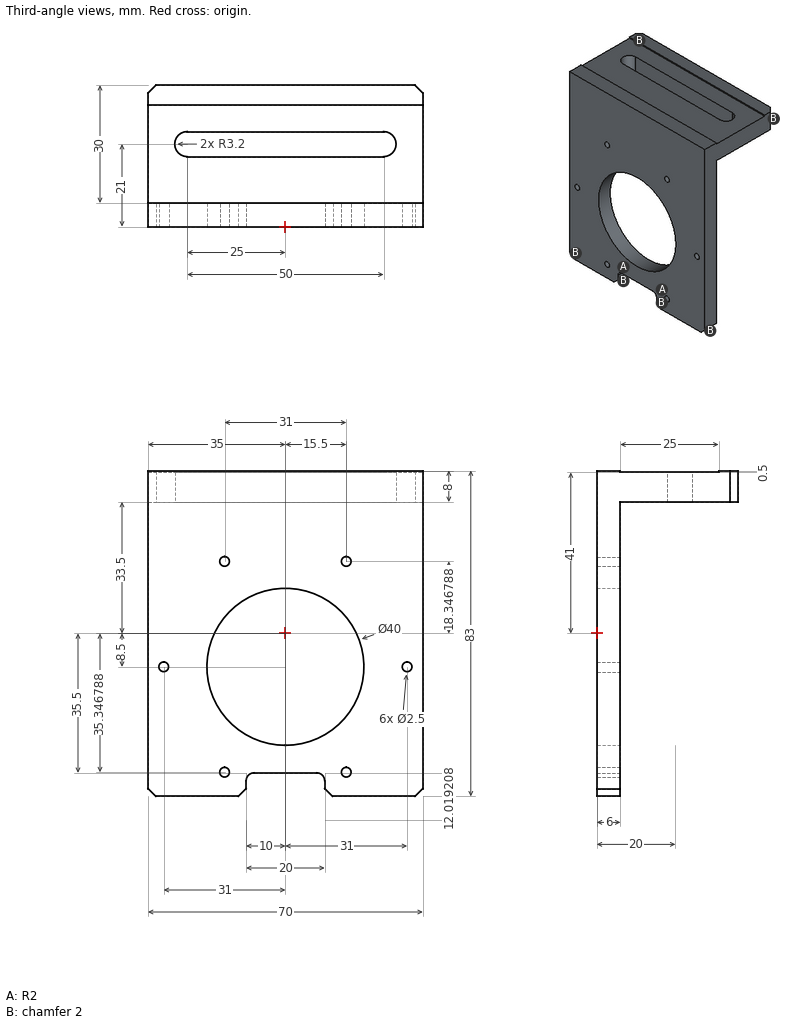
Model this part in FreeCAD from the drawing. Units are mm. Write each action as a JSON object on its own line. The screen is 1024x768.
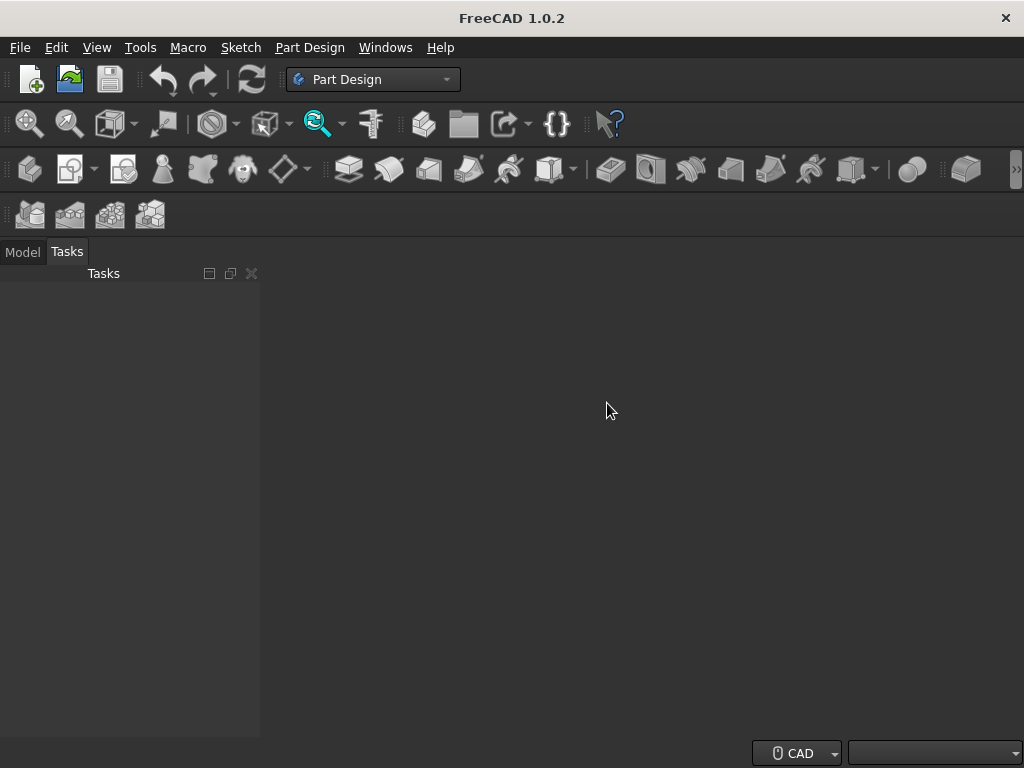
{"action": "left_click", "coordinate": [30, 80]}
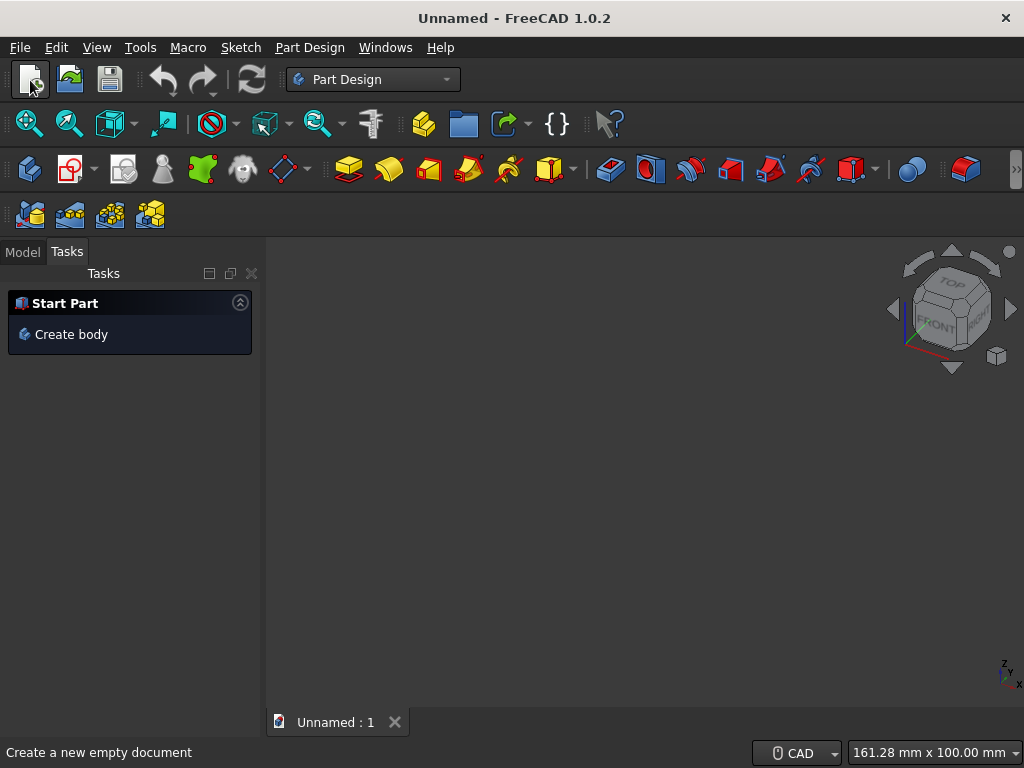
{"action": "left_click", "coordinate": [70, 170]}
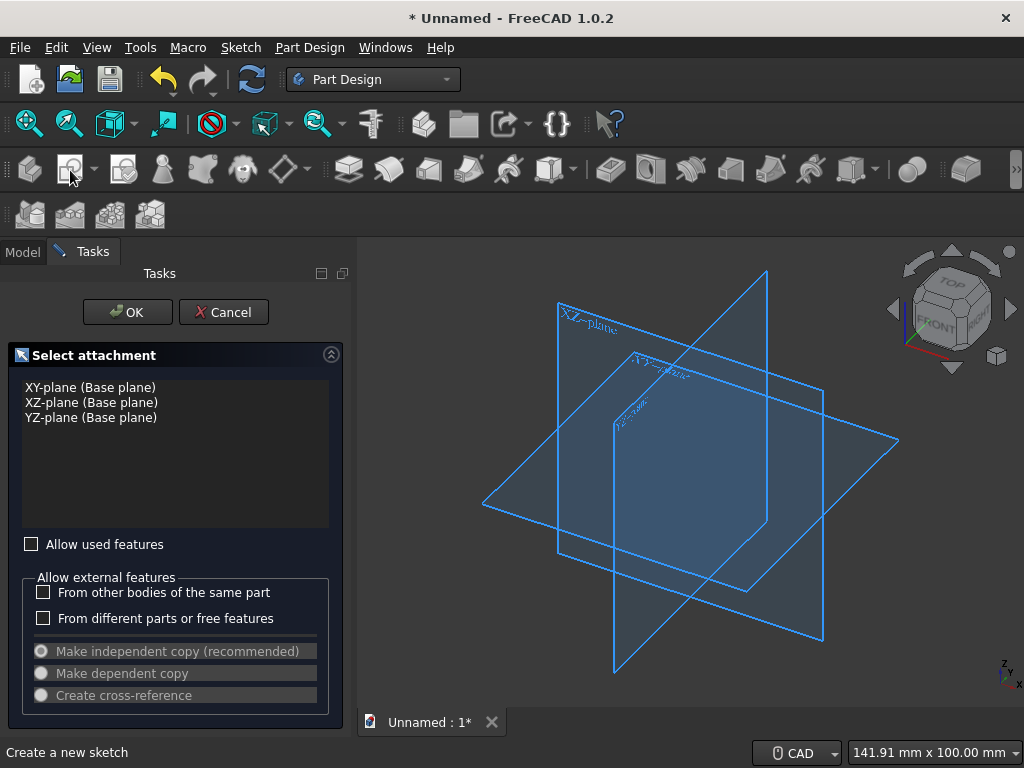
{"action": "left_click", "coordinate": [82, 402]}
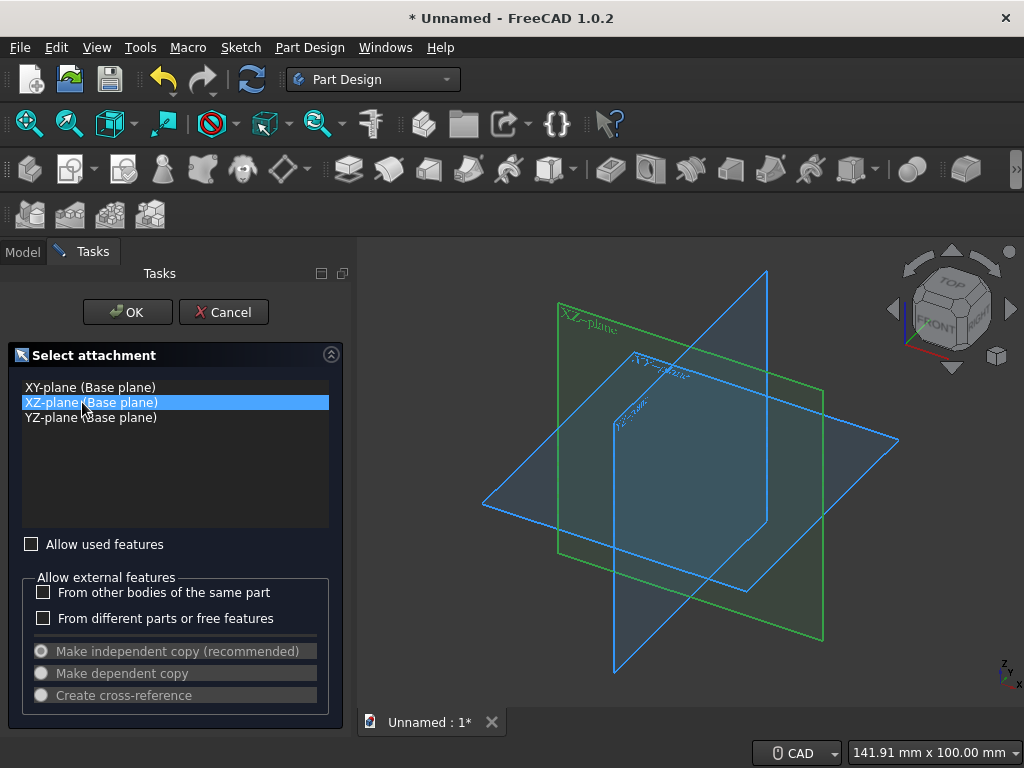
{"action": "left_click", "coordinate": [128, 312]}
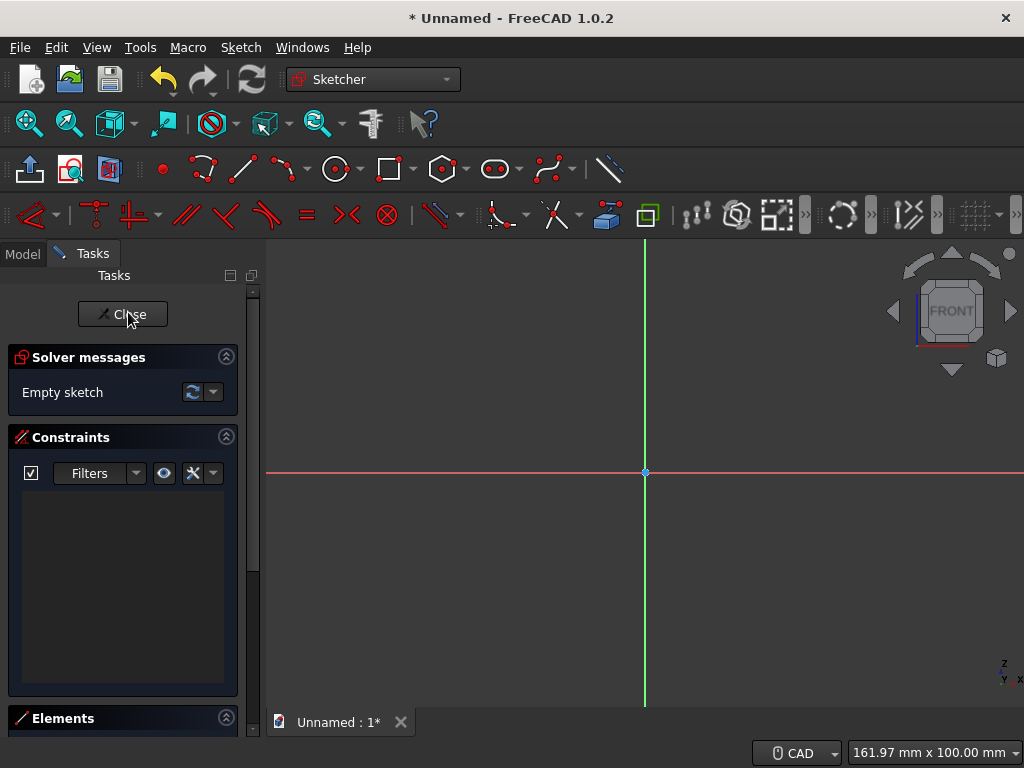
{"action": "scroll", "coordinate": [294, 473], "scroll_direction": "down", "scroll_amount": 1}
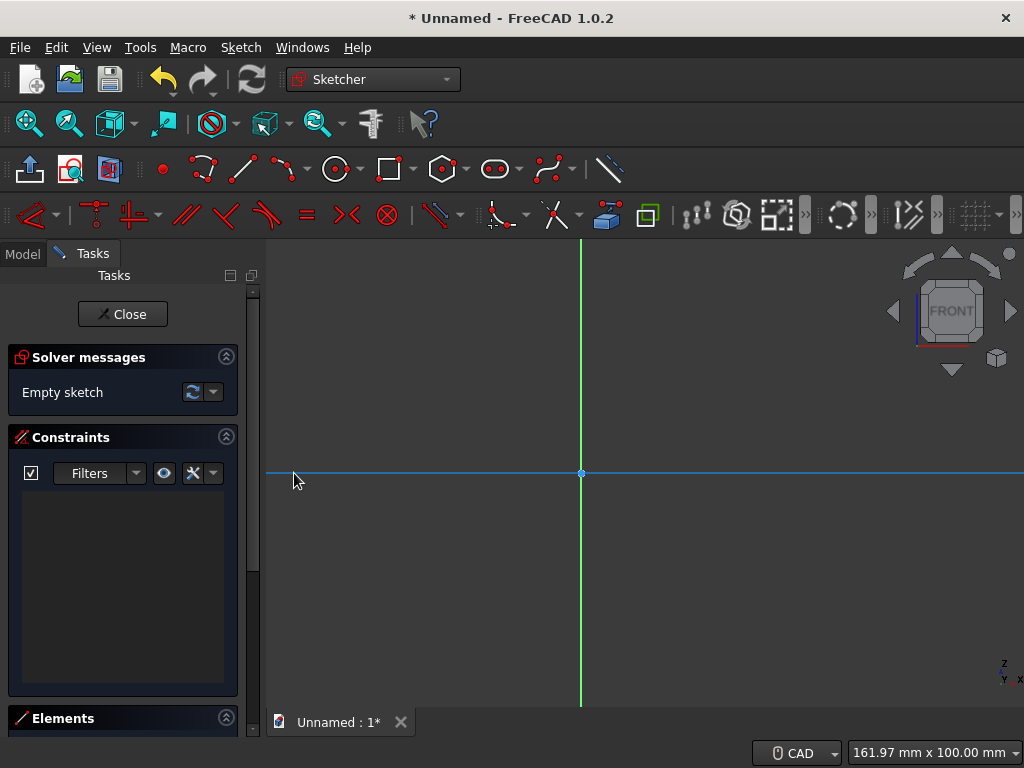
{"action": "left_click", "coordinate": [416, 170]}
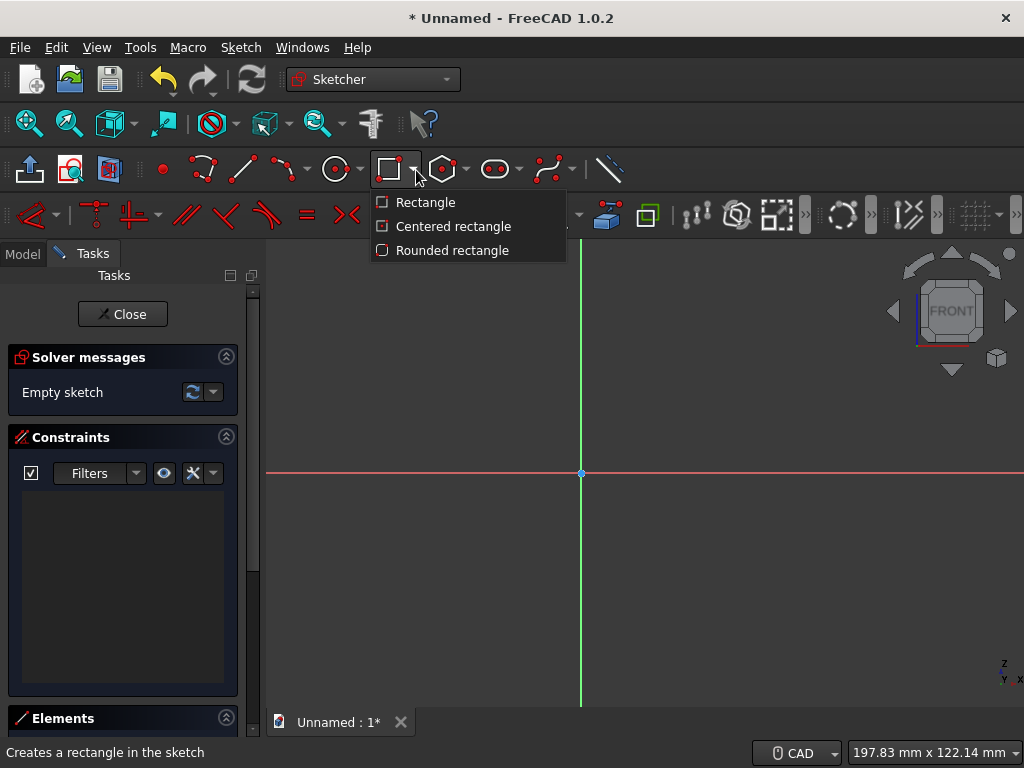
{"action": "left_click", "coordinate": [468, 226]}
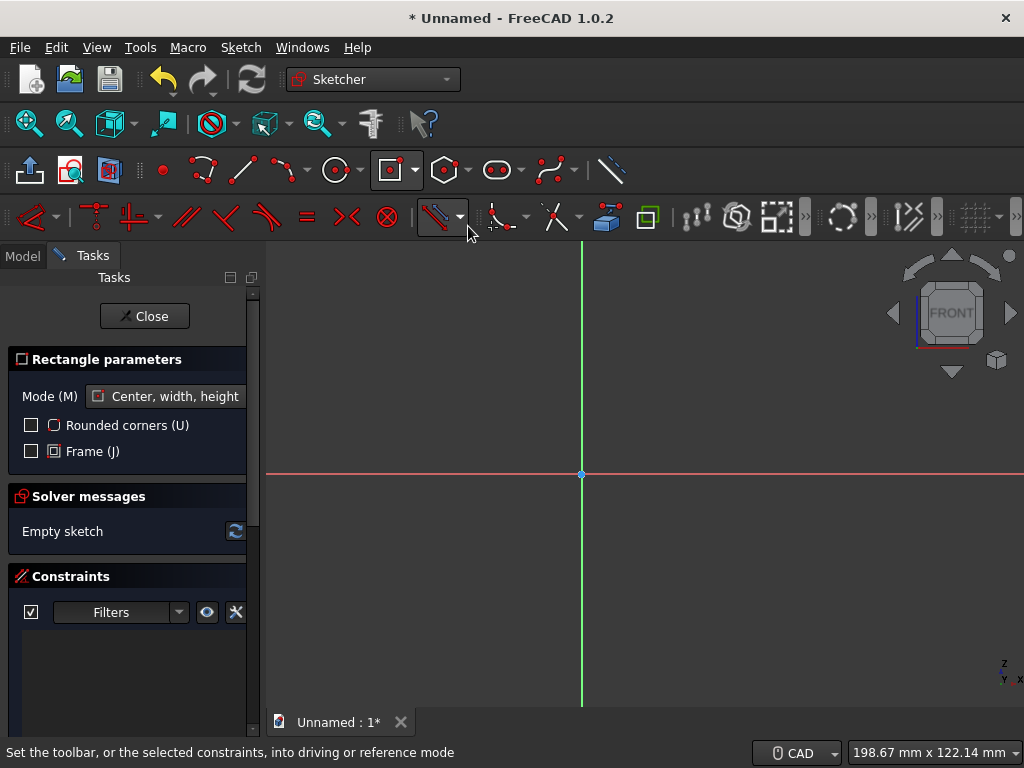
{"action": "left_click", "coordinate": [582, 474]}
{"action": "mouse_move", "coordinate": [715, 316]}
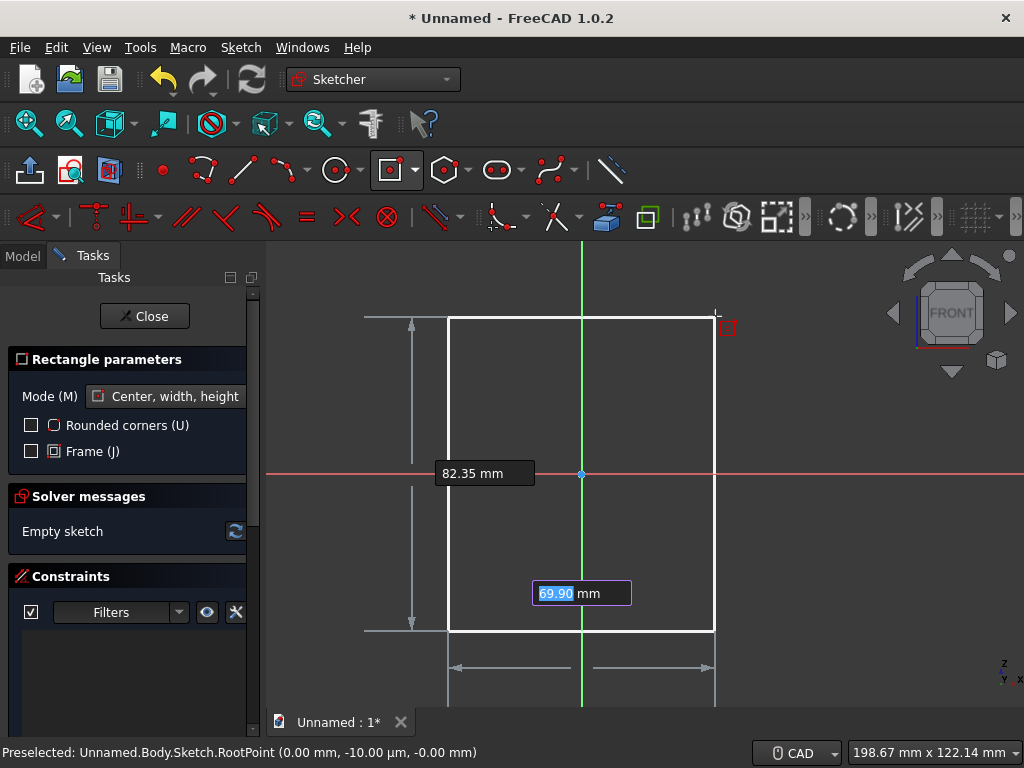
{"action": "type", "text": "70"}
{"action": "key", "text": "Tab"}
{"action": "type", "text": "83"}
{"action": "key", "text": "Return"}
{"action": "key", "text": "Escape"}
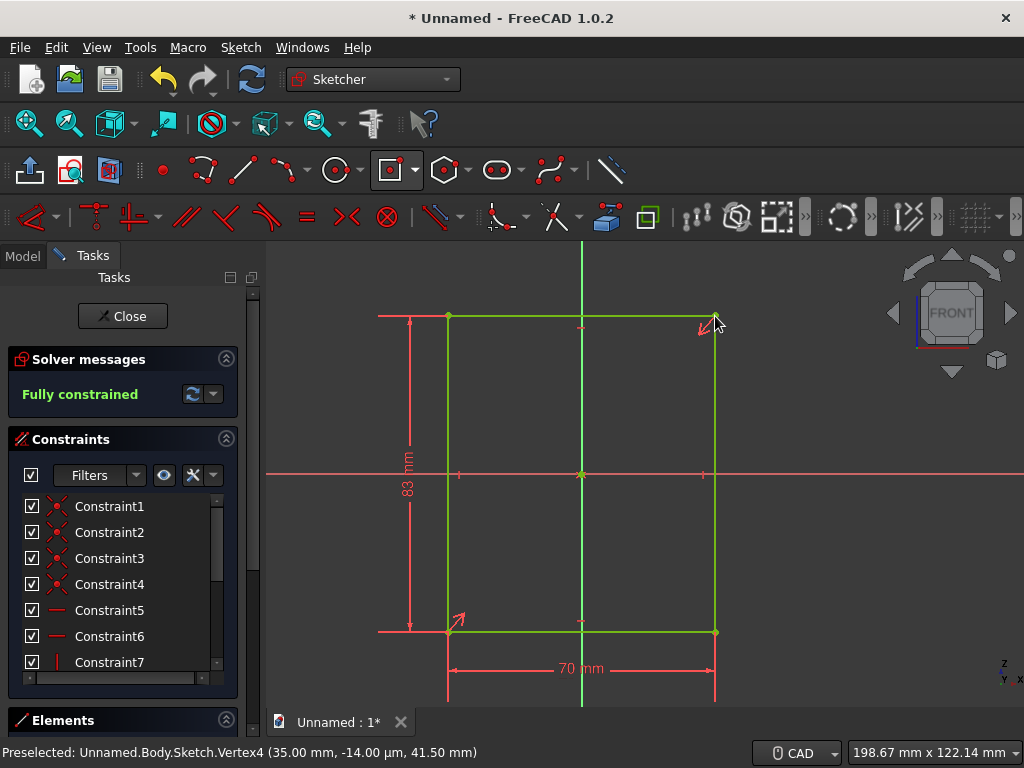
{"action": "left_click", "coordinate": [123, 316]}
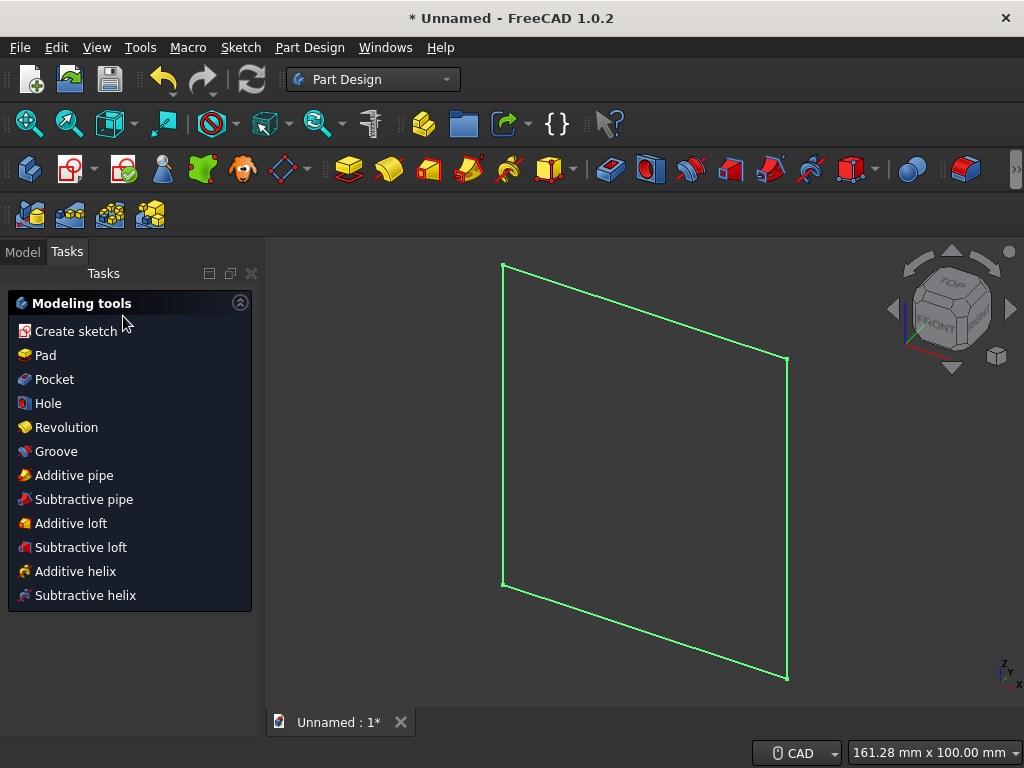
{"action": "left_click", "coordinate": [350, 170]}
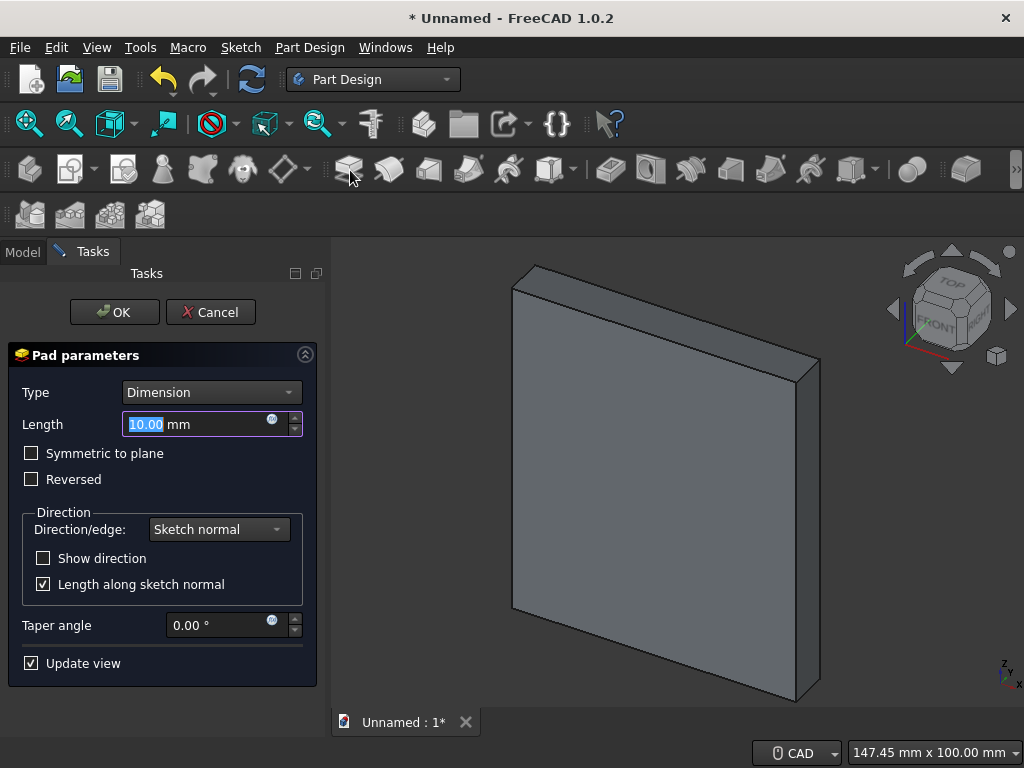
{"action": "type", "text": "6"}
{"action": "key", "text": "Tab"}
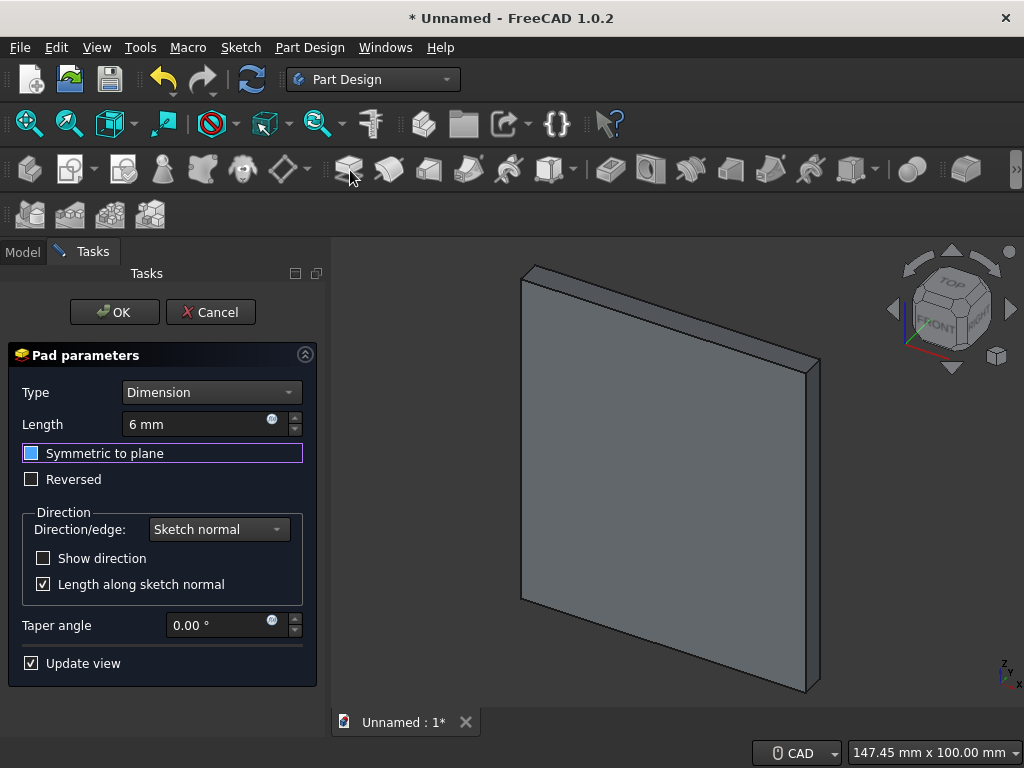
{"action": "left_click", "coordinate": [30, 479]}